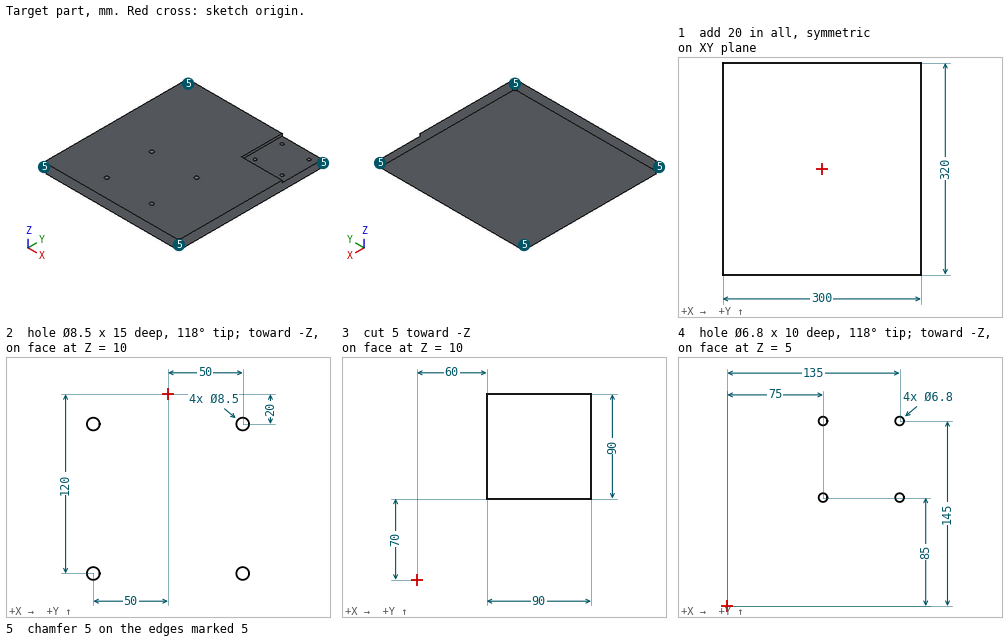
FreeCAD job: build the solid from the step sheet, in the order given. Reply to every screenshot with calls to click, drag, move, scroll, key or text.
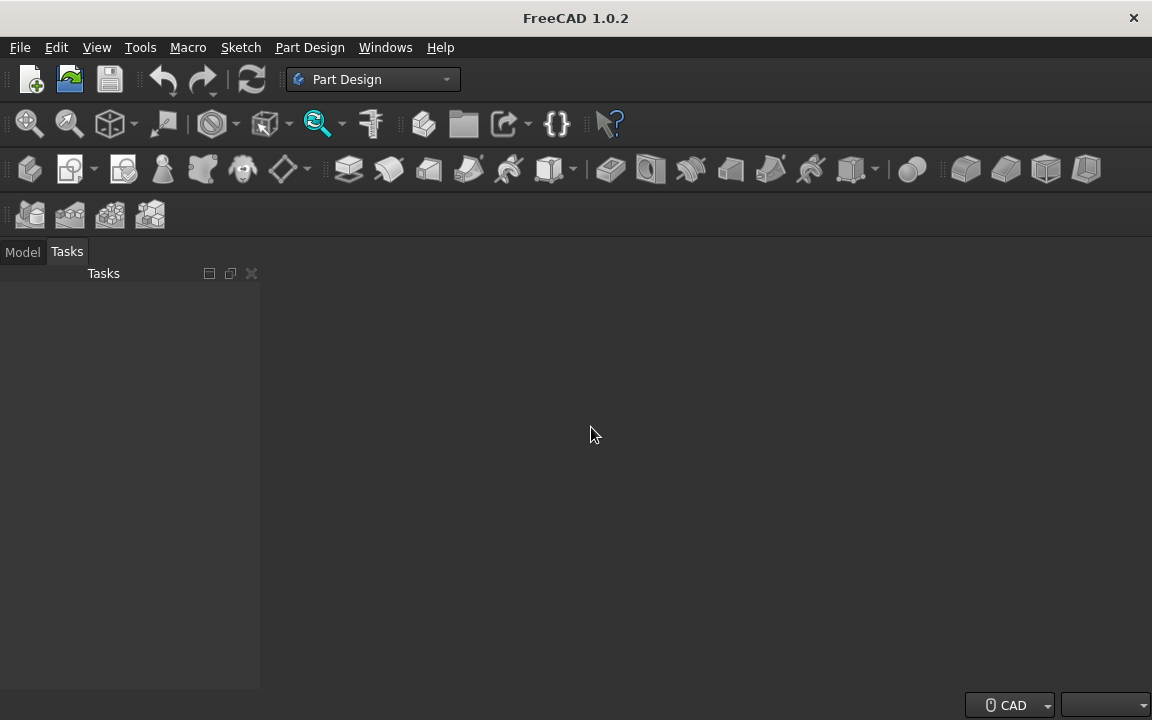
key(ctrl+n)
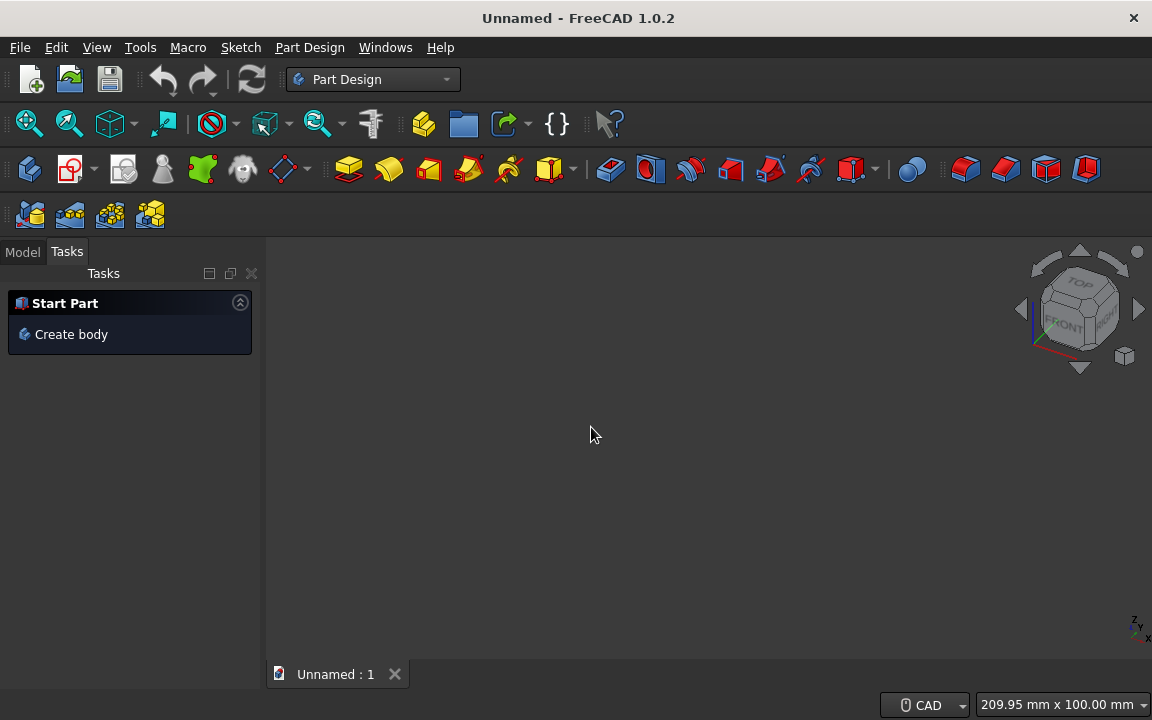
click(70, 170)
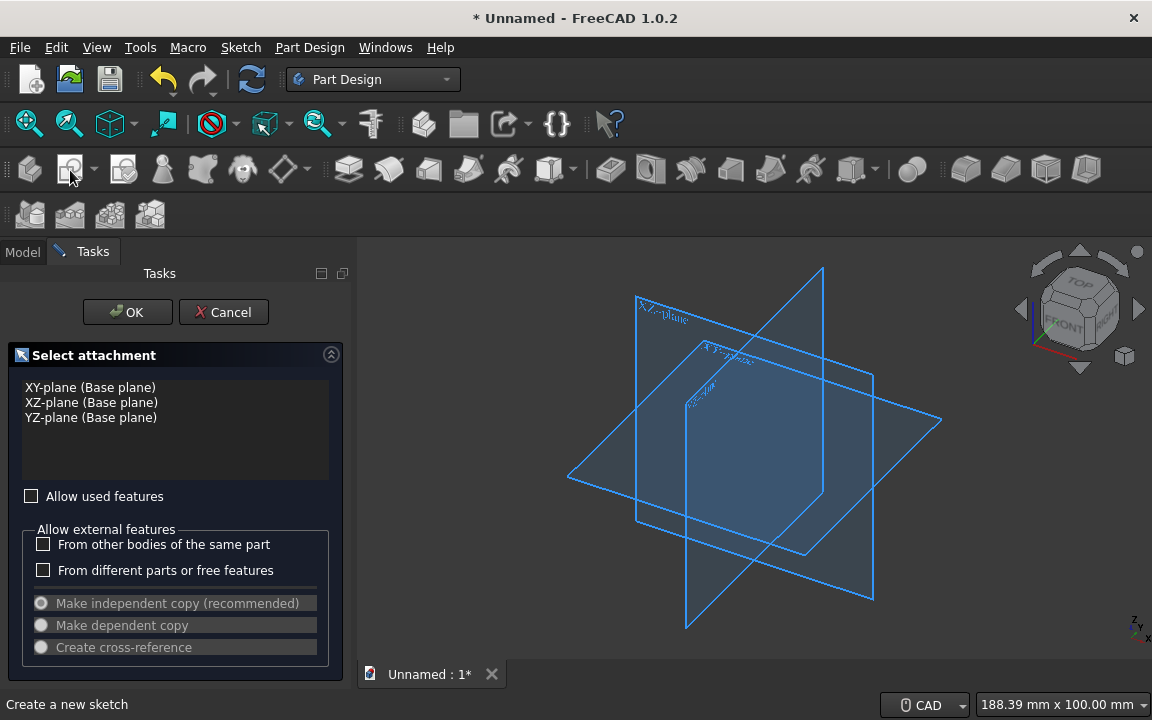
click(82, 388)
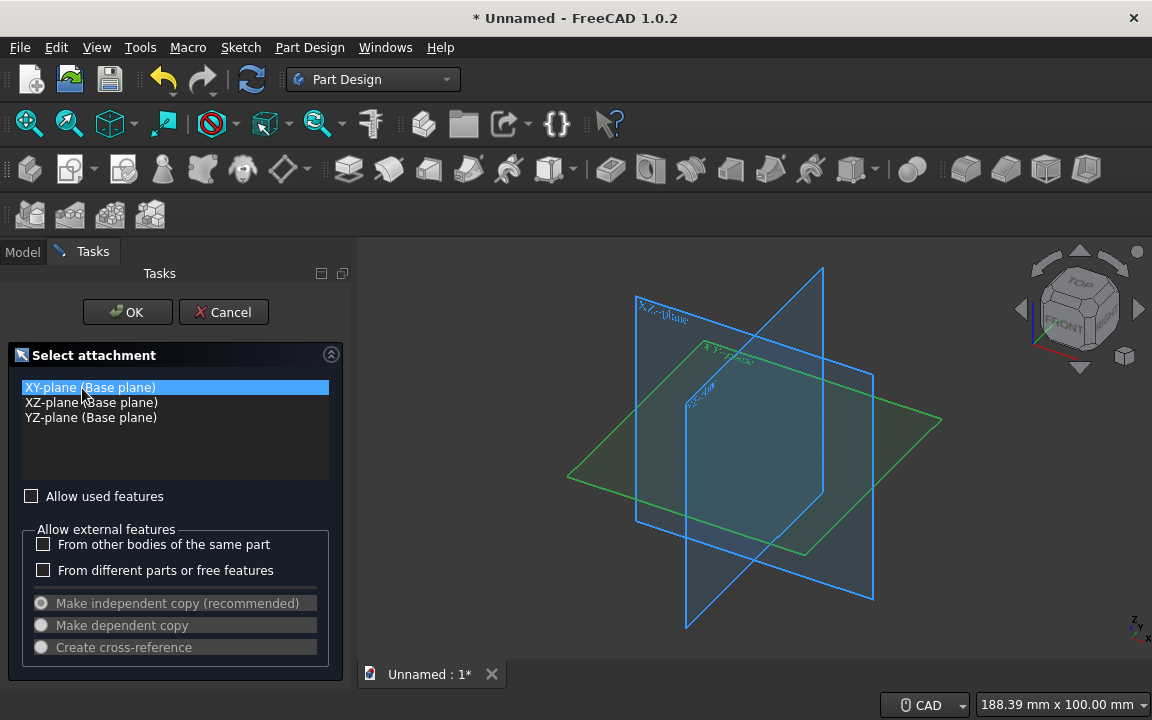
click(128, 312)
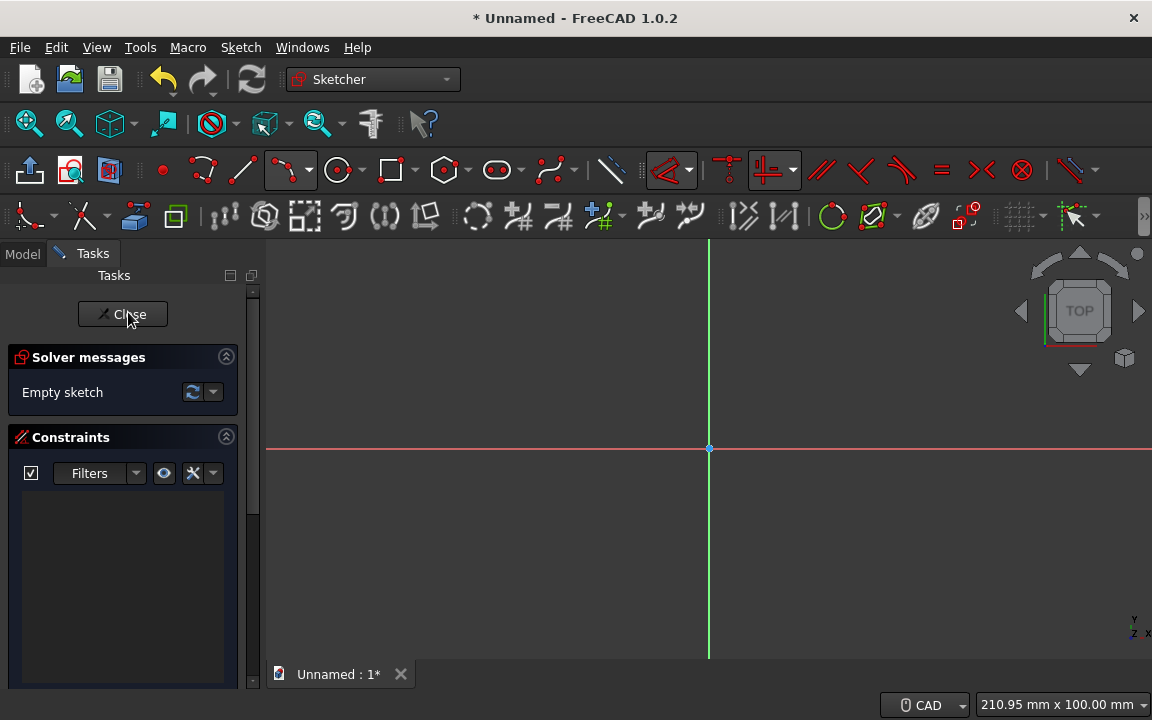
scroll(623, 449, down, 8)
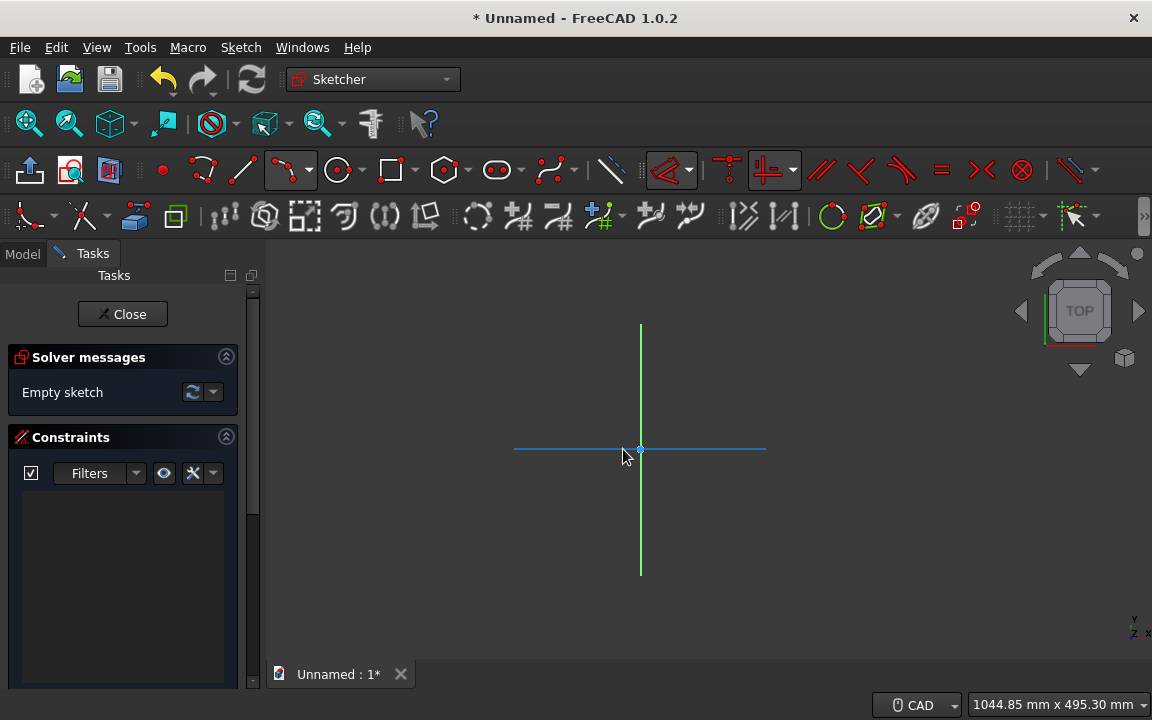
key(g)
key(v)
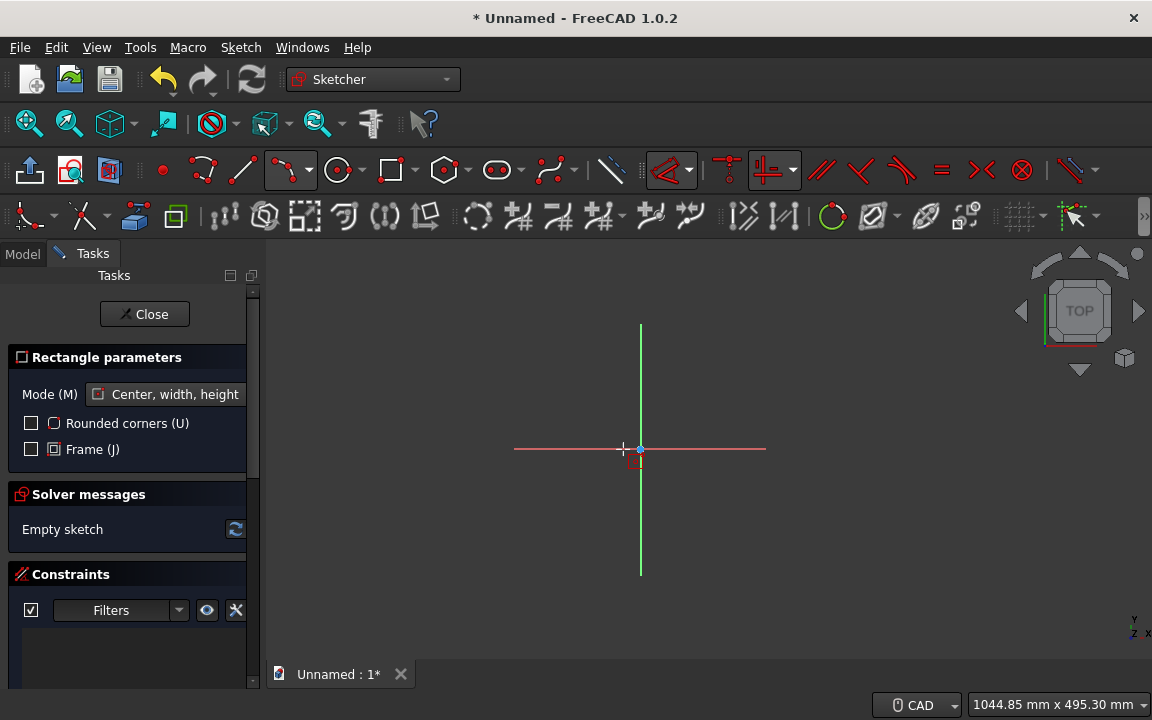
click(641, 449)
move(768, 314)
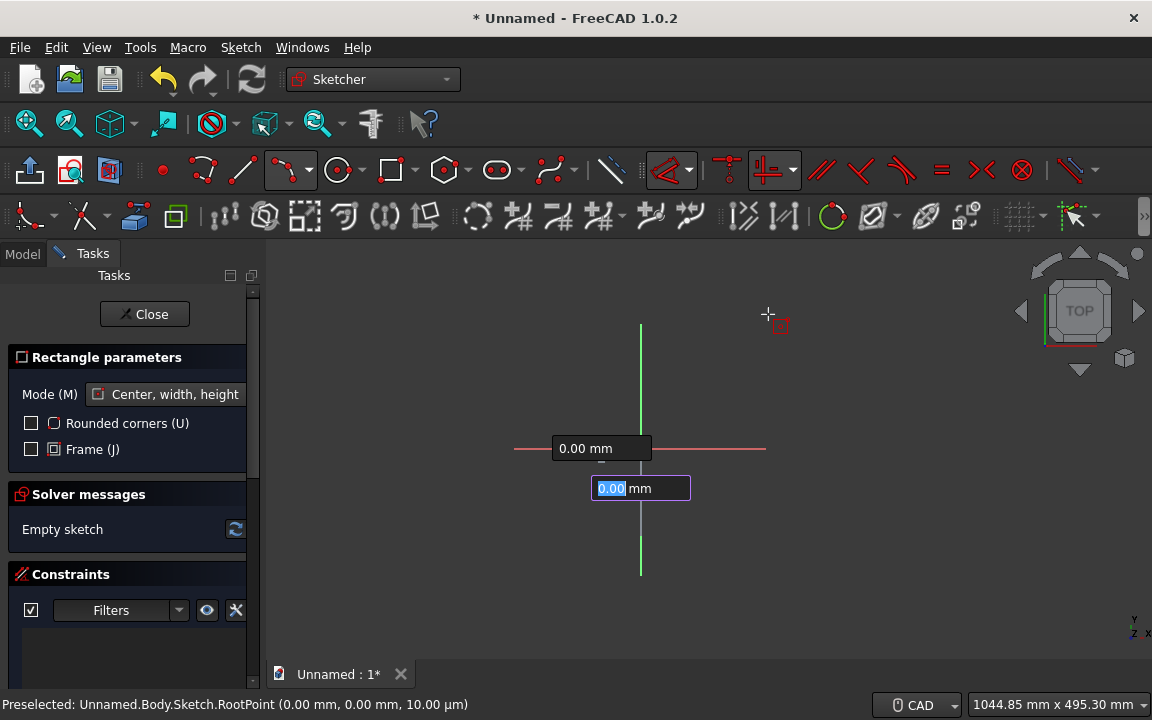
text(300)
key(Tab)
text(320)
key(Return)
key(Escape)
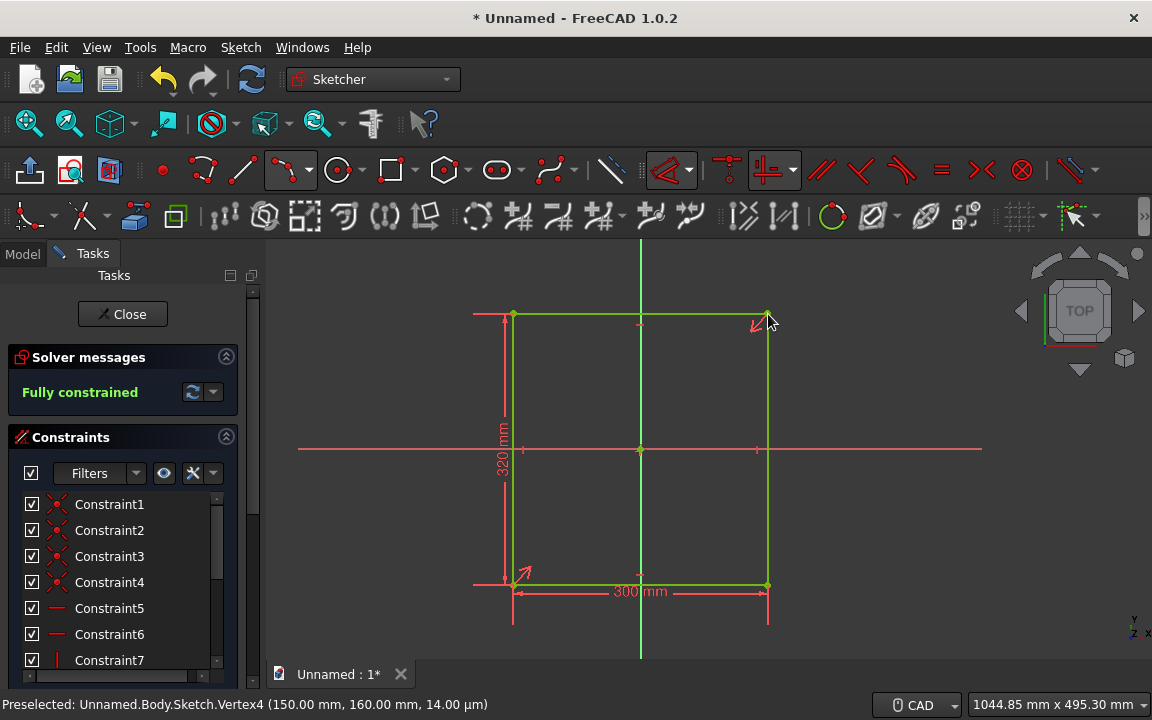
click(123, 314)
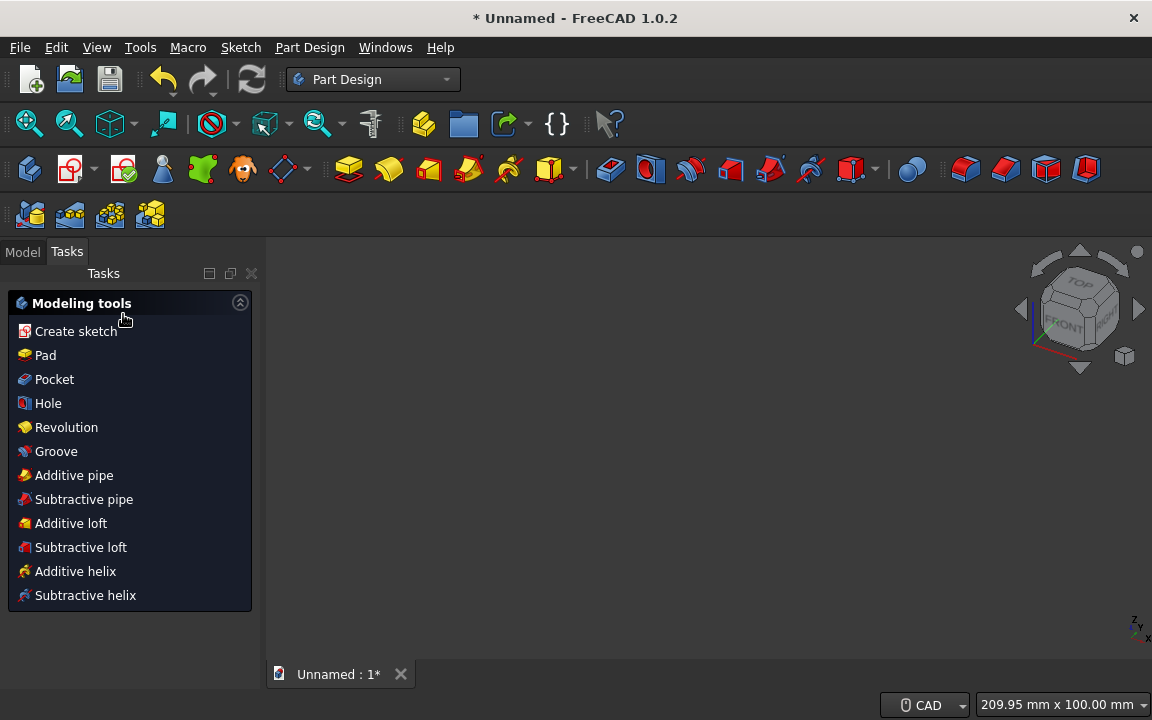
click(350, 170)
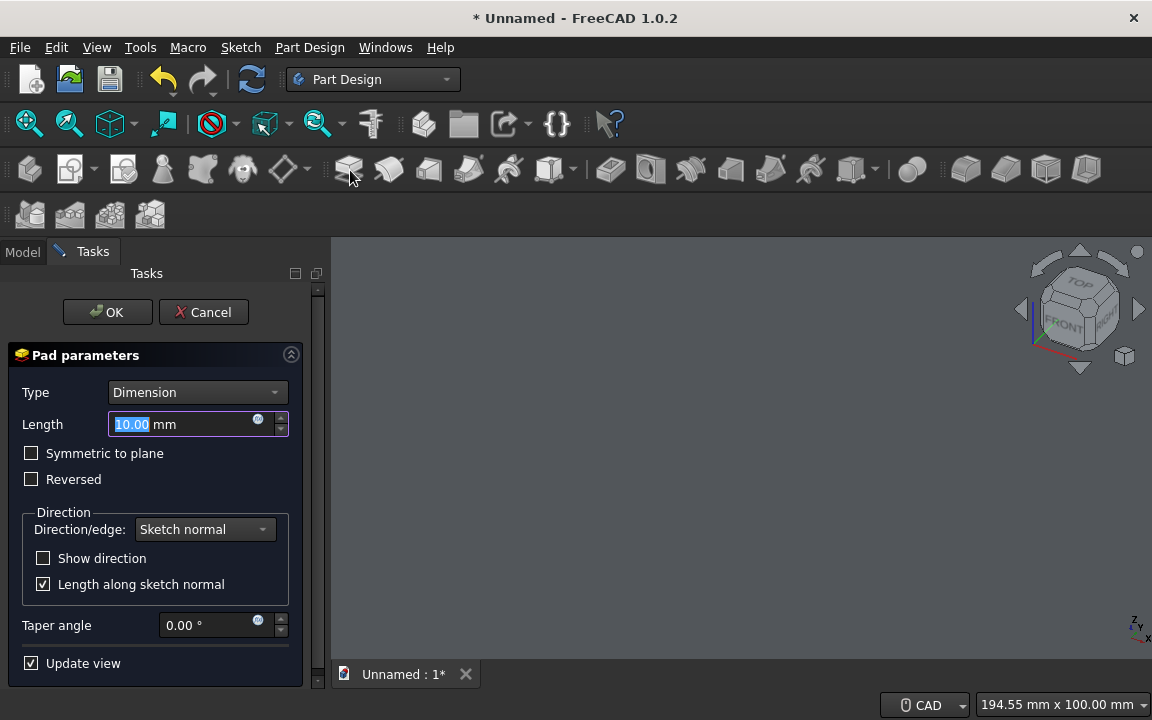
text(20)
key(Tab)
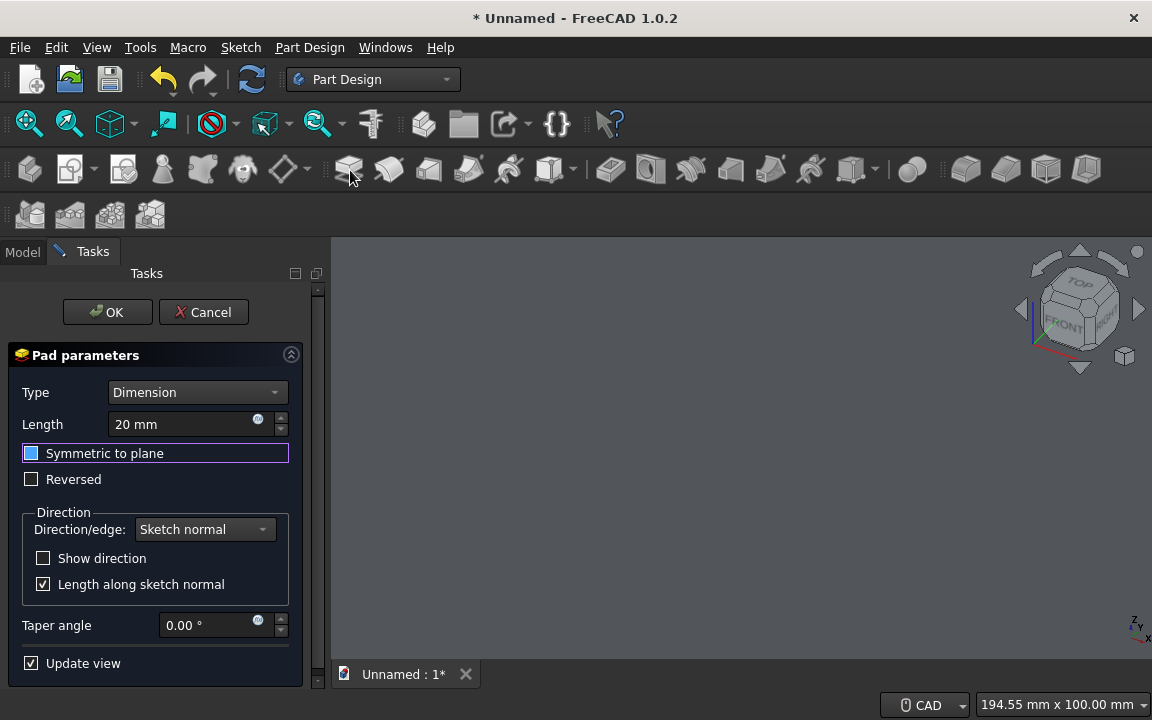
click(30, 453)